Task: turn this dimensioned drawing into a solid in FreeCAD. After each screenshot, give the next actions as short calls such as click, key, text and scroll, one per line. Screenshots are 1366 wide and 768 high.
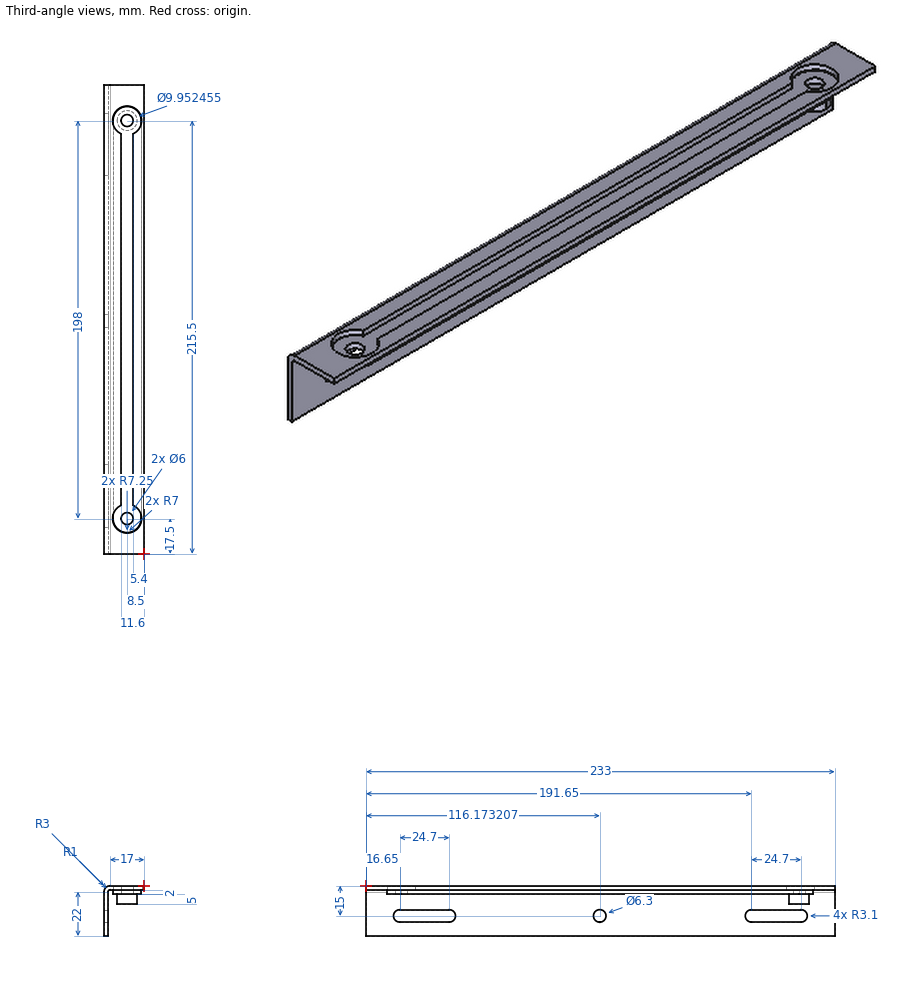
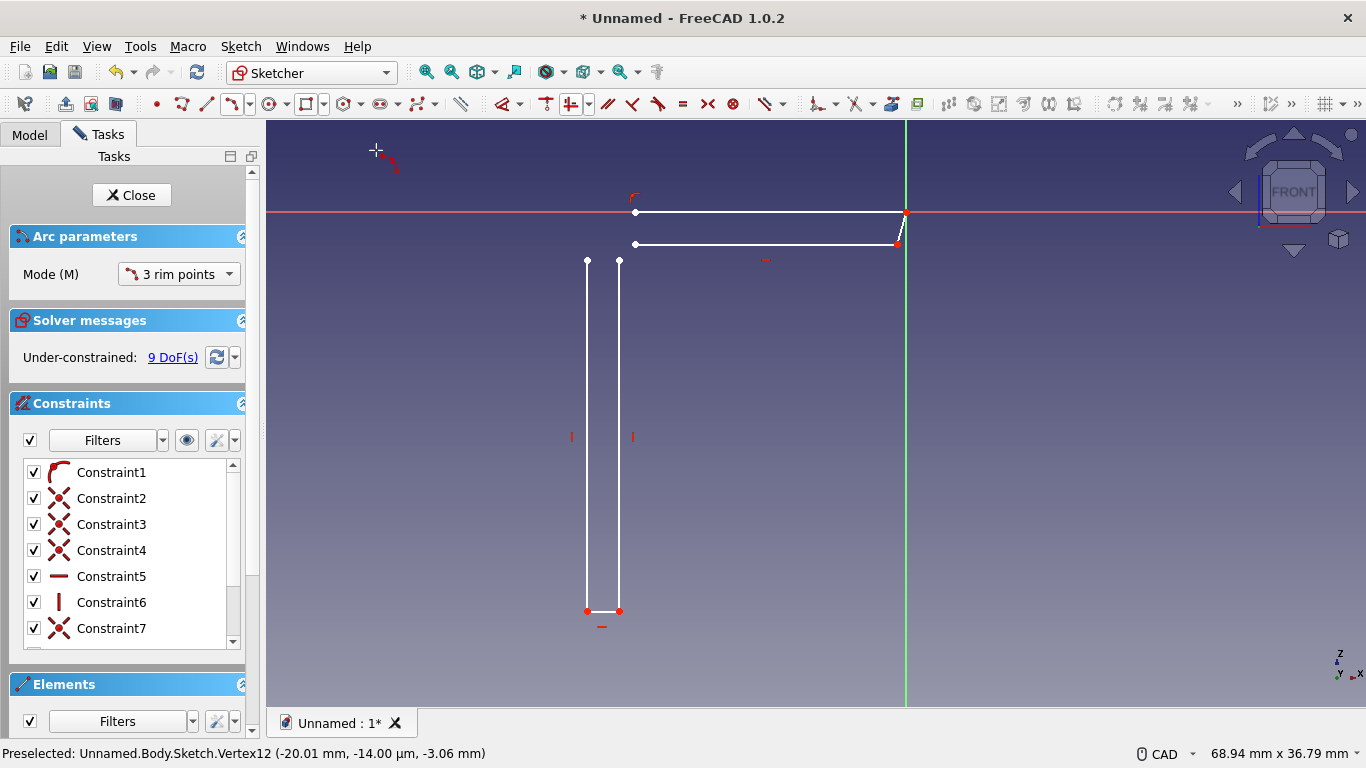
click(635, 245)
click(619, 261)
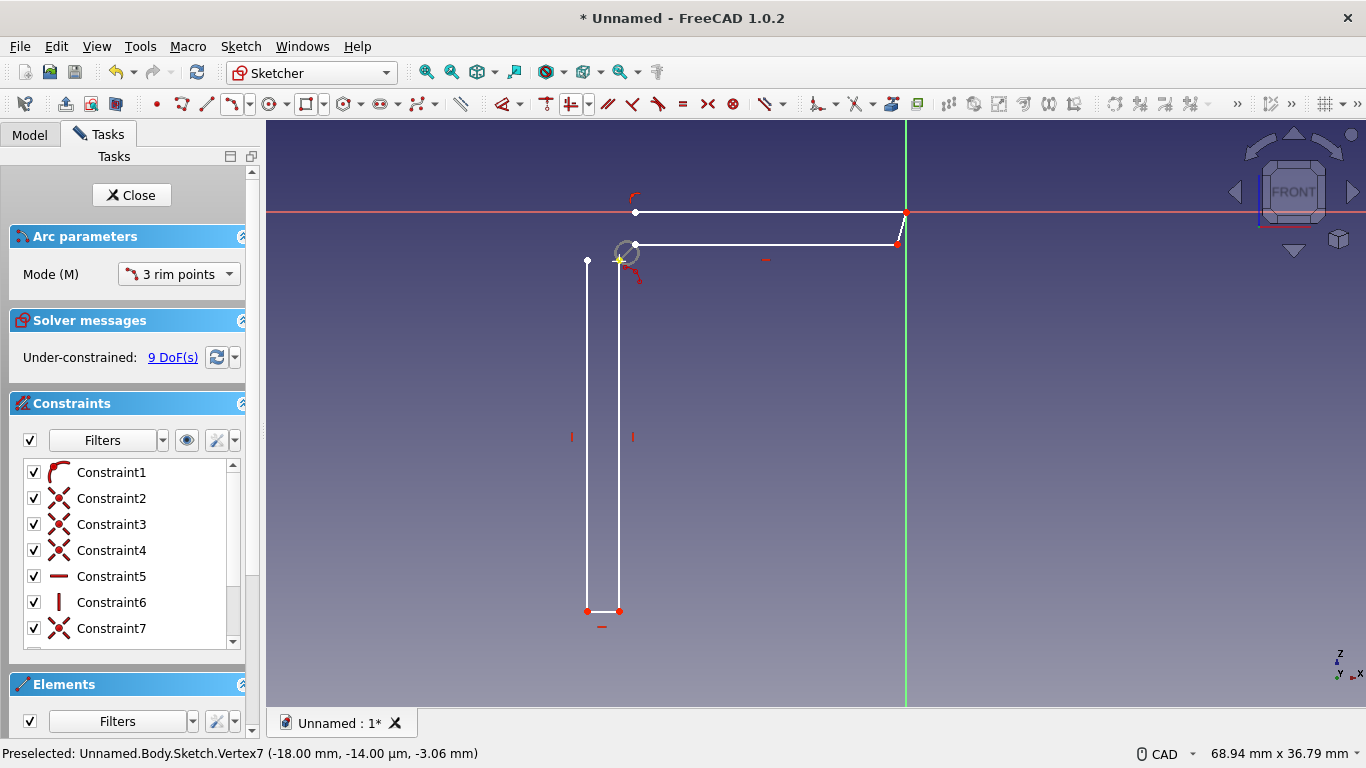
scroll(624, 249, up, 7)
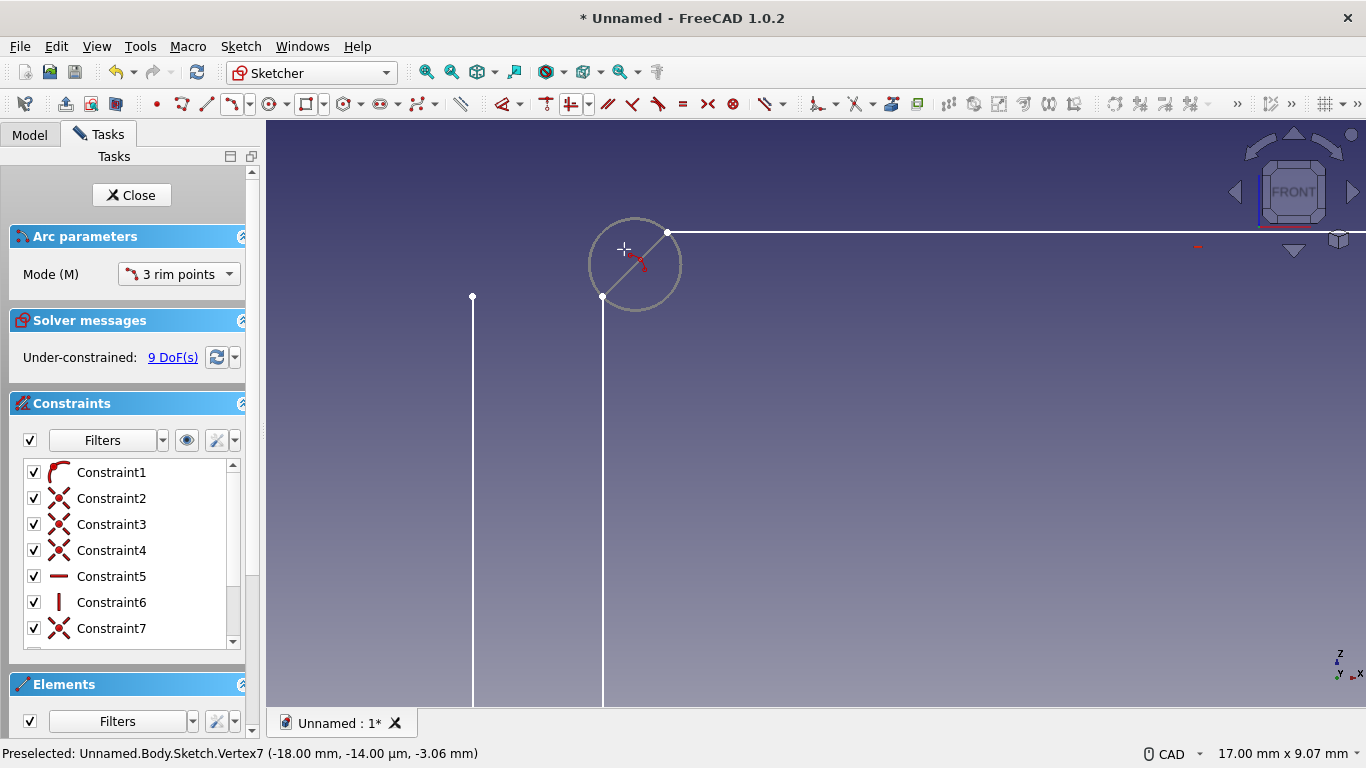
click(622, 247)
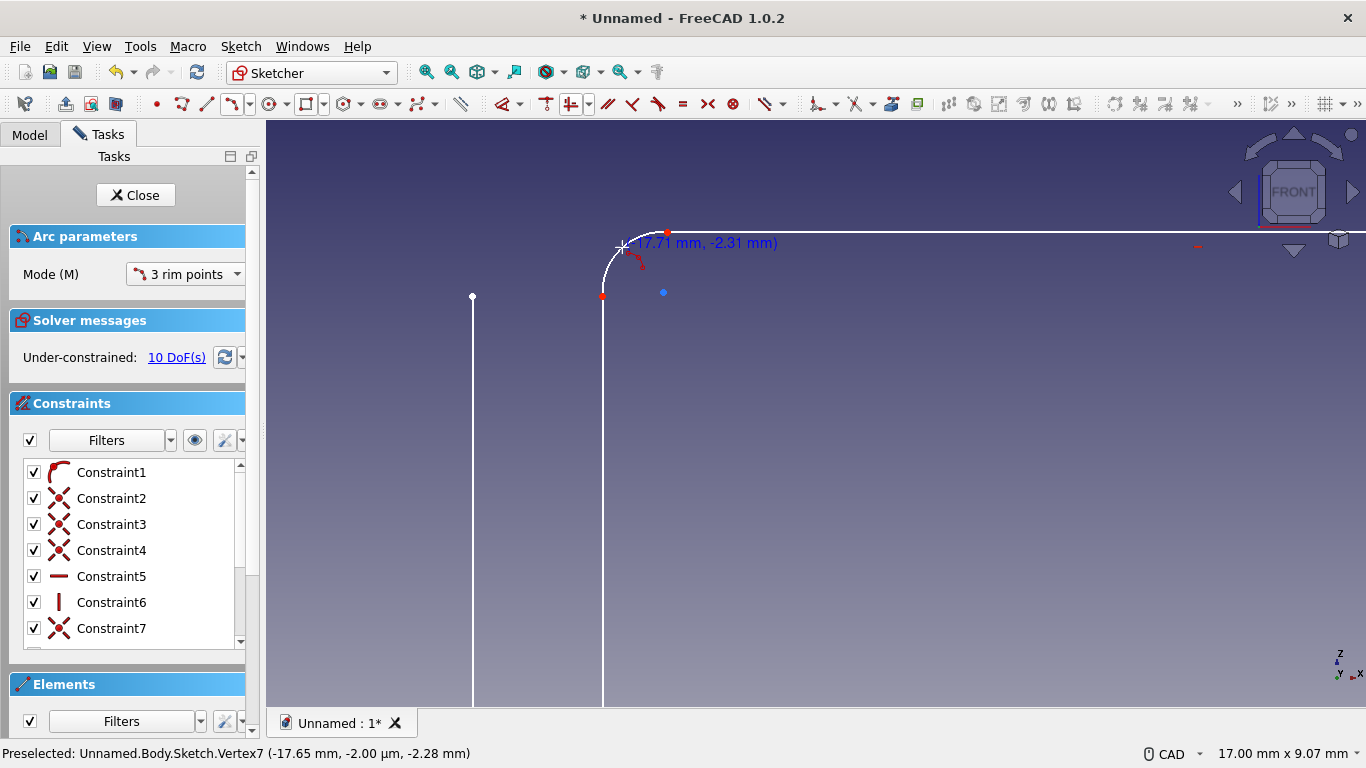
scroll(625, 252, down, 7)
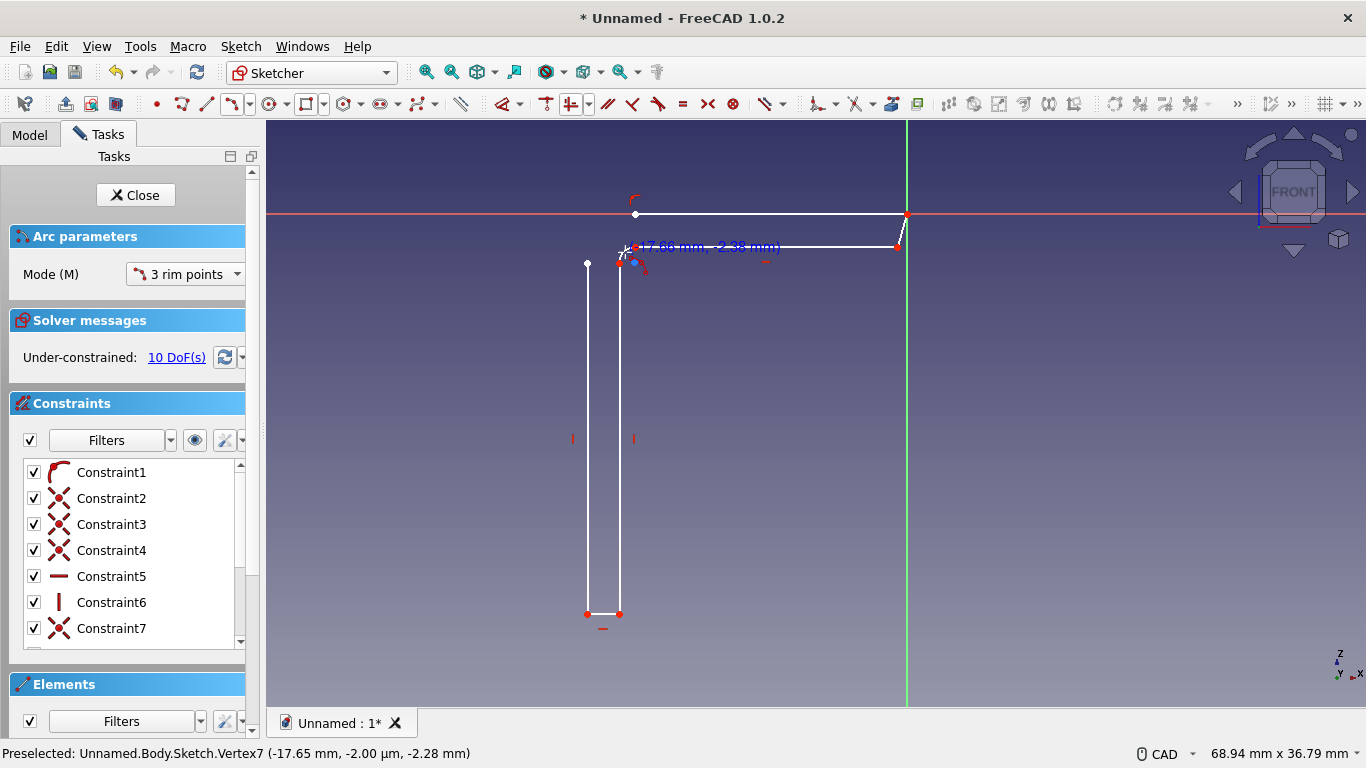
click(588, 263)
click(636, 214)
click(602, 228)
key(Escape)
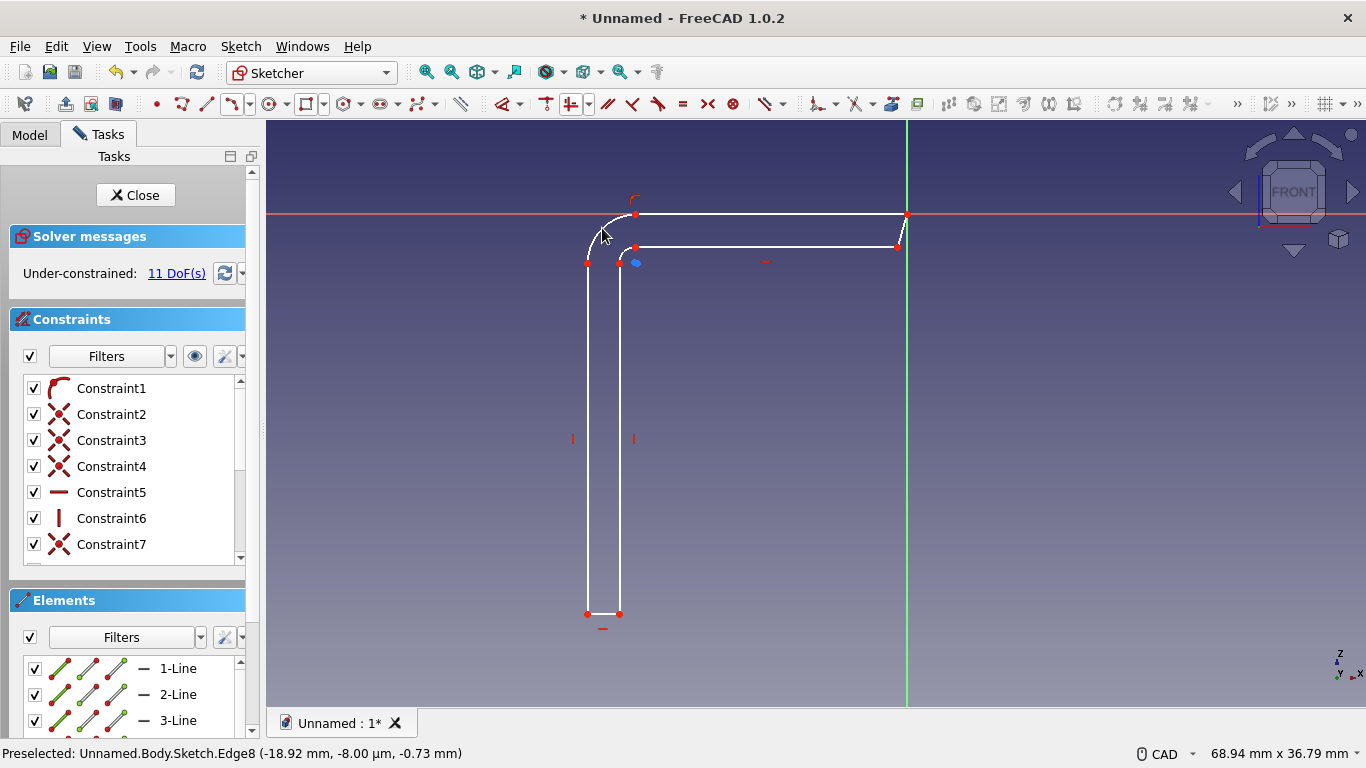
click(717, 214)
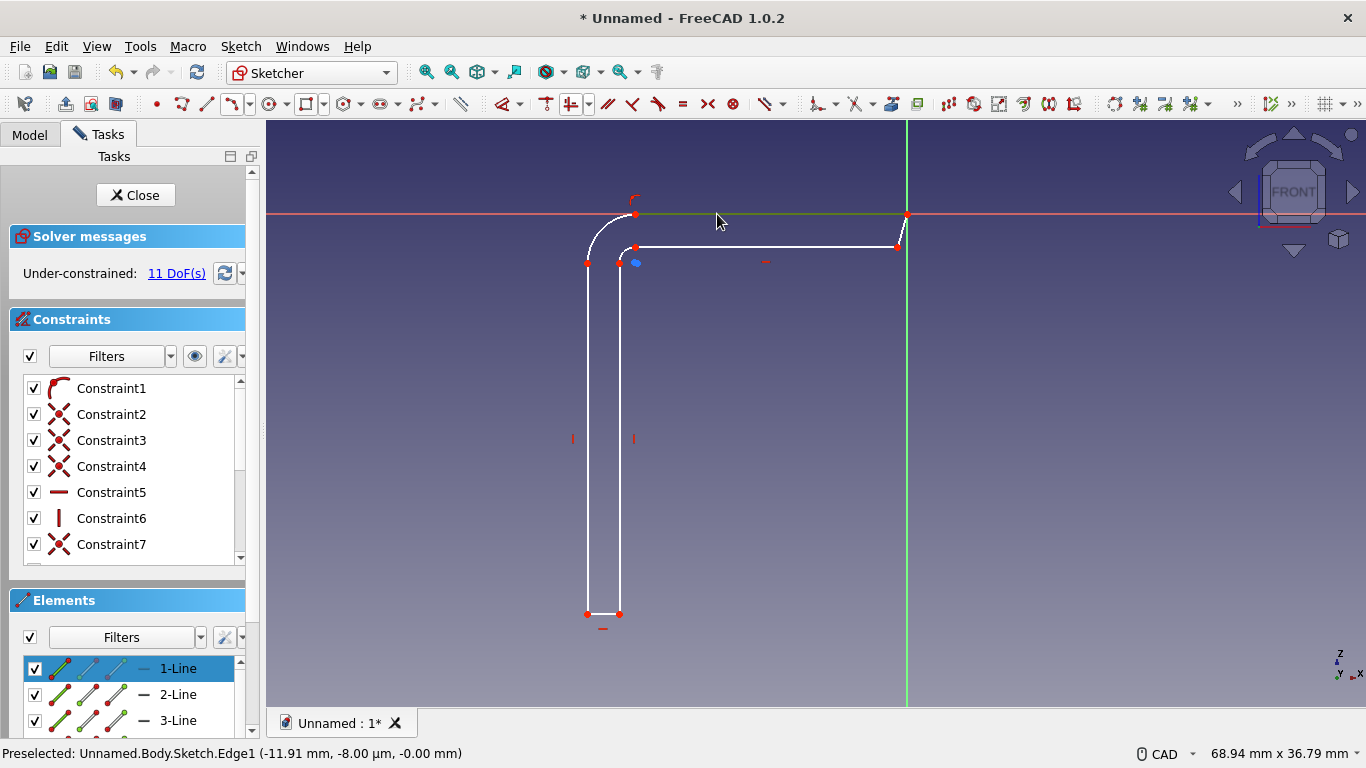
click(593, 241)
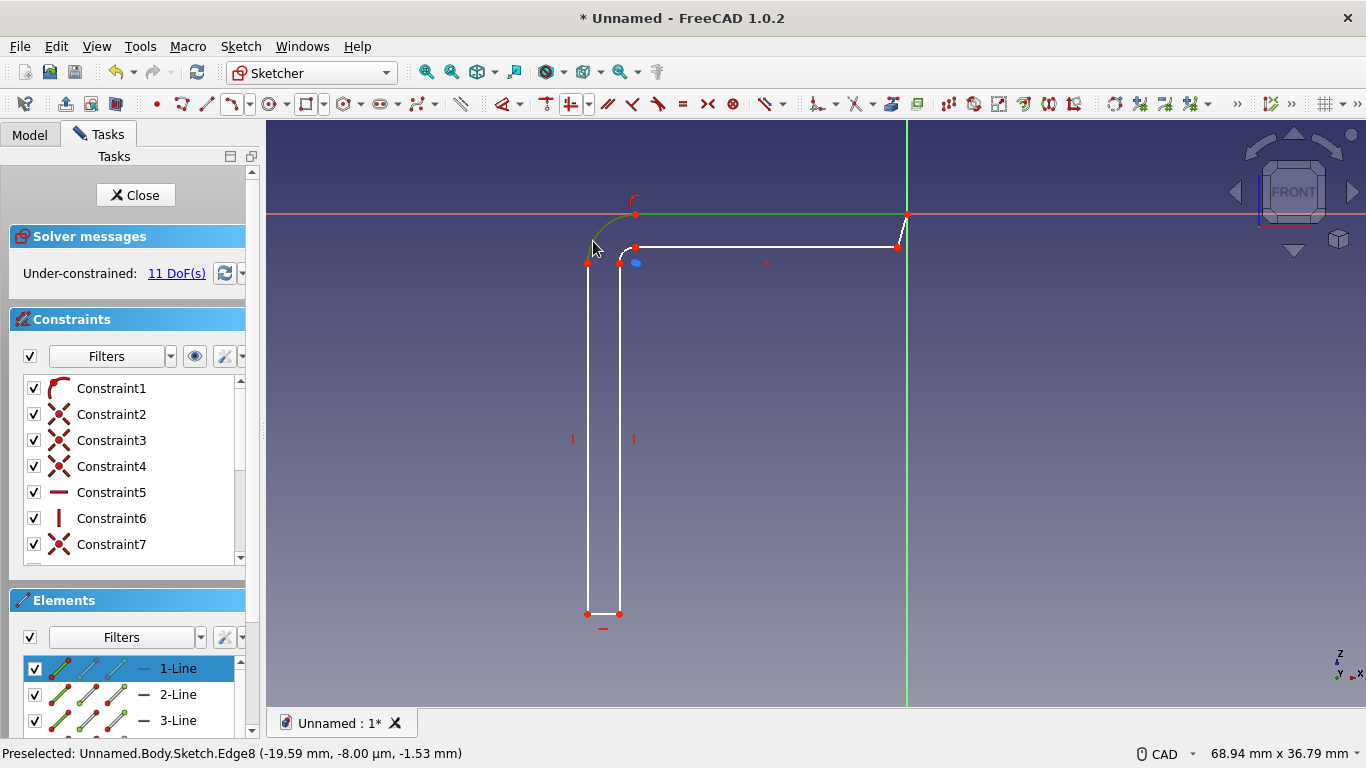
click(658, 104)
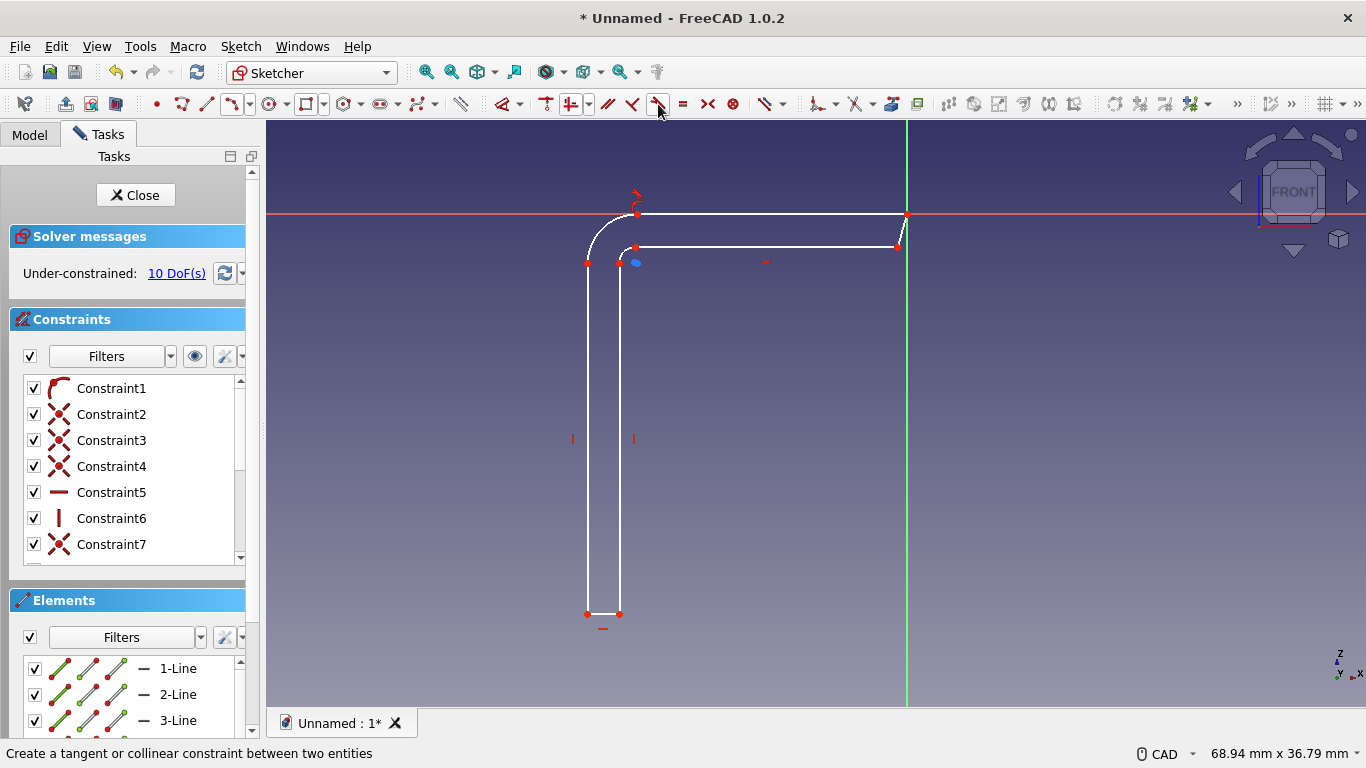
click(819, 247)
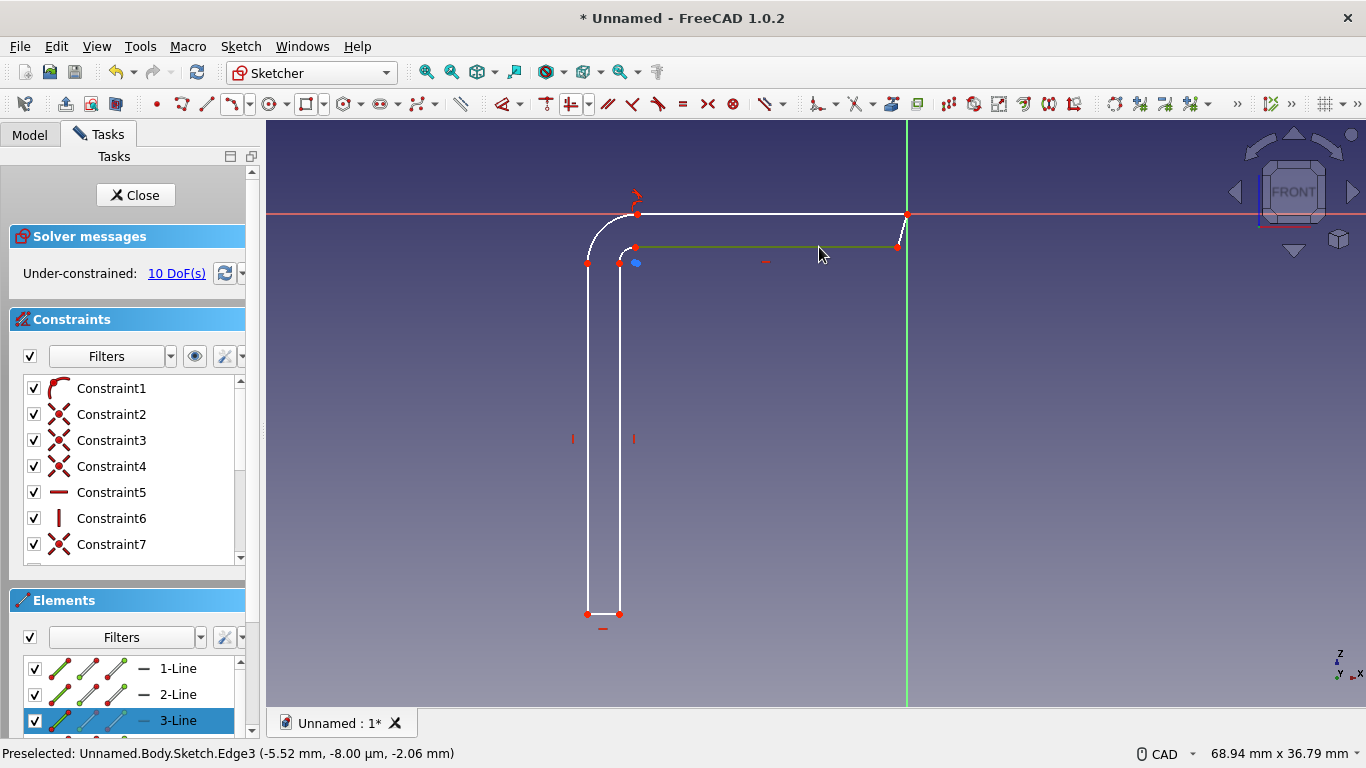
click(624, 252)